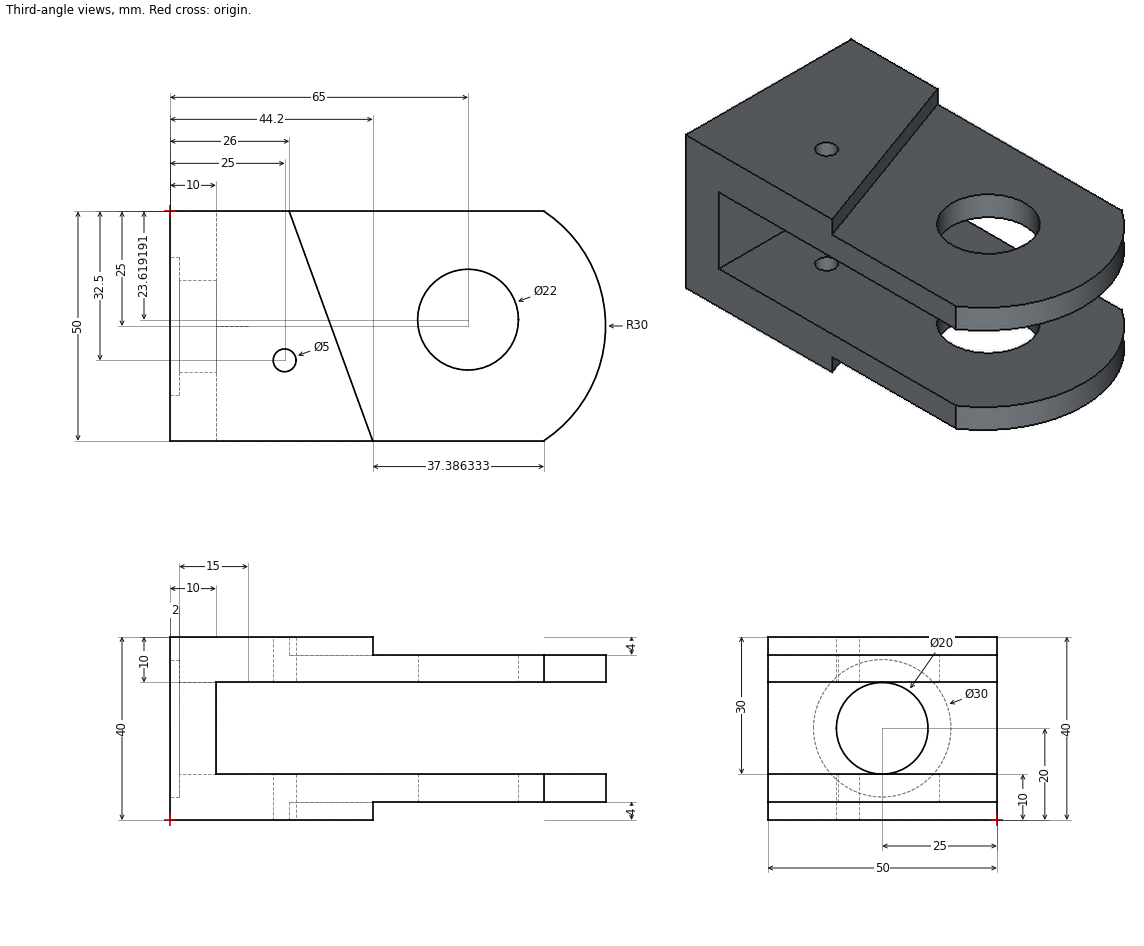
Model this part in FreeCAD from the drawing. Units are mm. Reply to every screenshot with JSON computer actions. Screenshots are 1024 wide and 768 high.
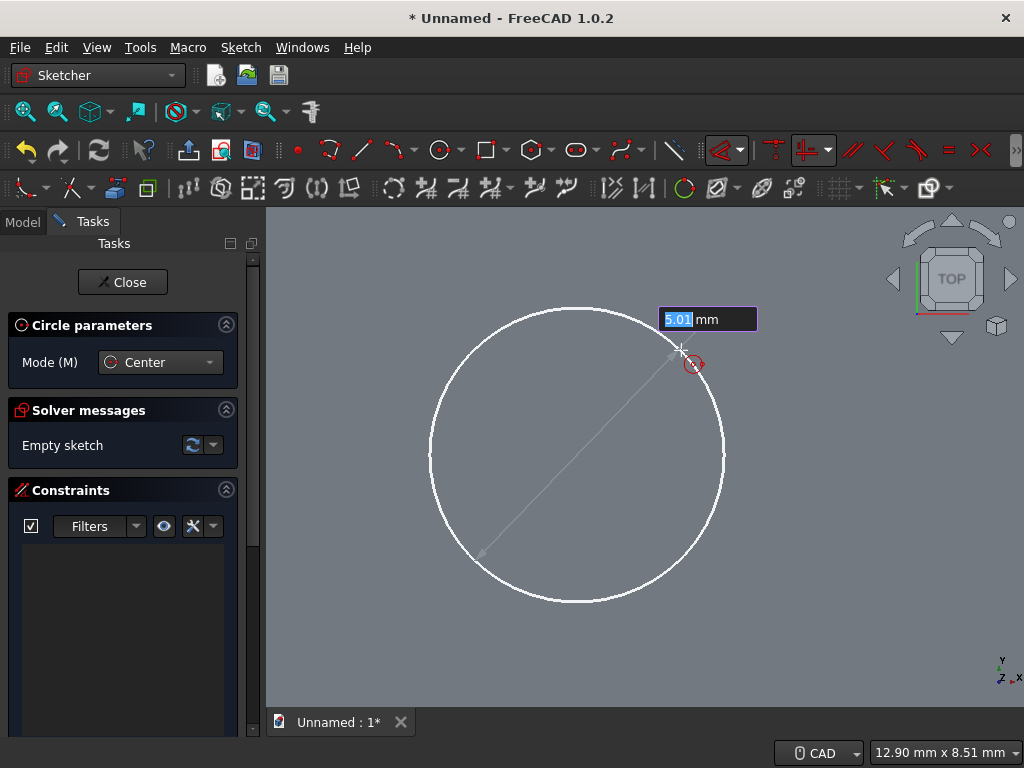
{"action": "type", "text": "5"}
{"action": "key", "text": "Return"}
{"action": "key", "text": "Escape"}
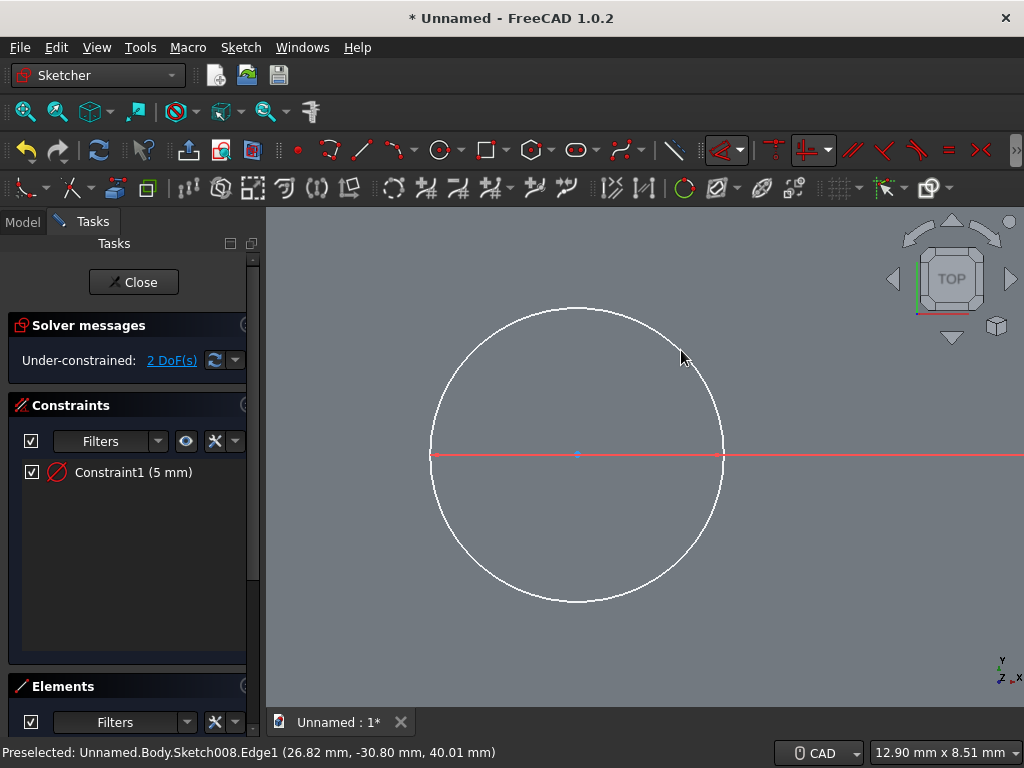
{"action": "left_click", "coordinate": [577, 455]}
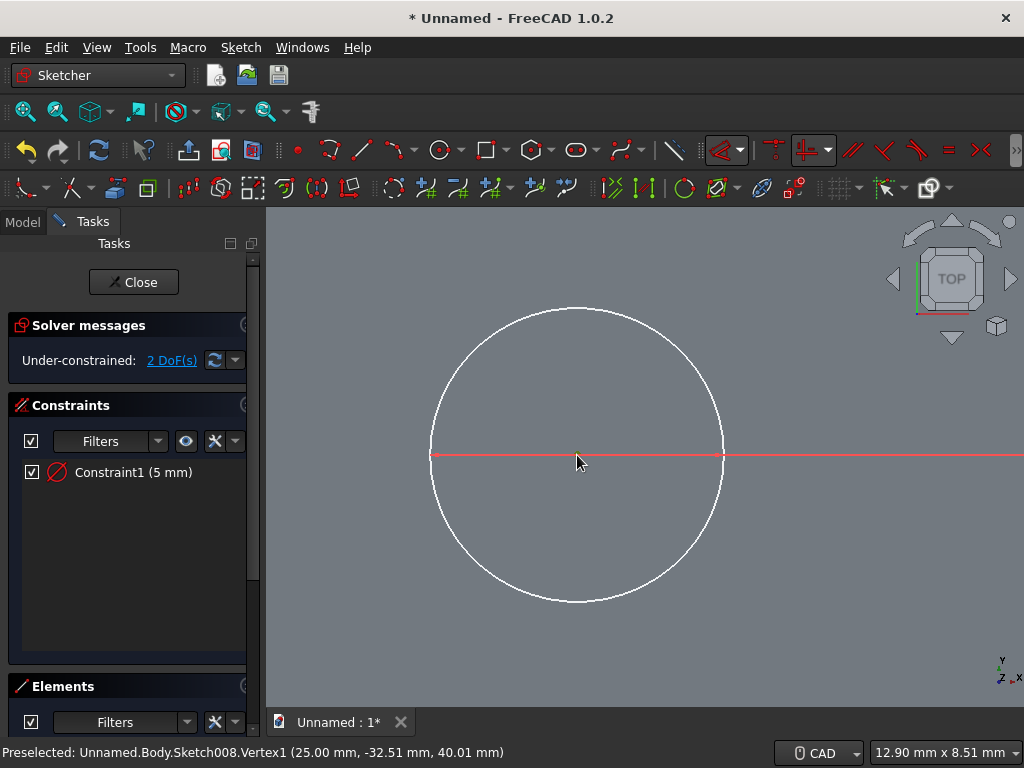
{"action": "key", "text": "l"}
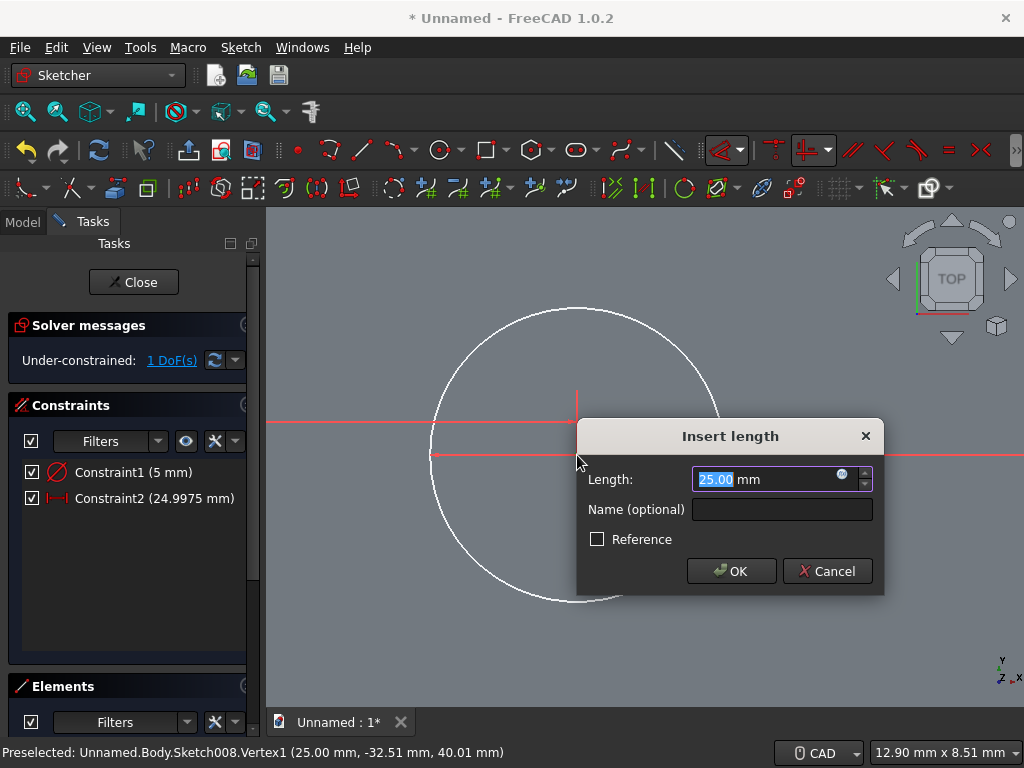
{"action": "type", "text": "25"}
{"action": "key", "text": "Return"}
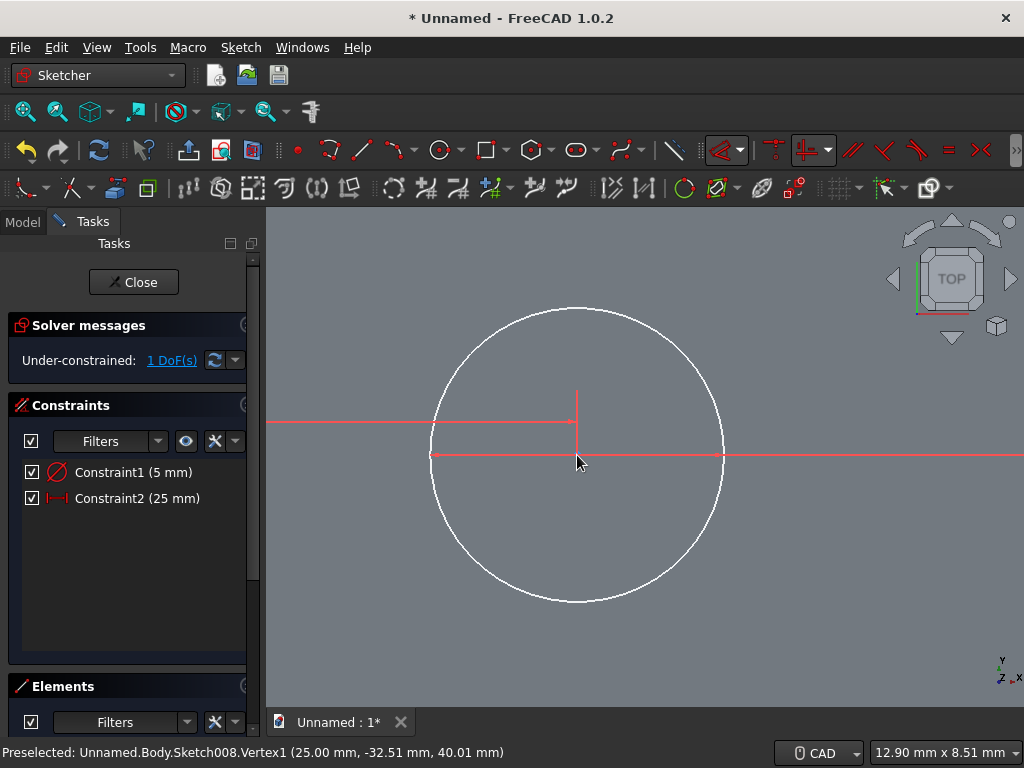
{"action": "left_click", "coordinate": [577, 455]}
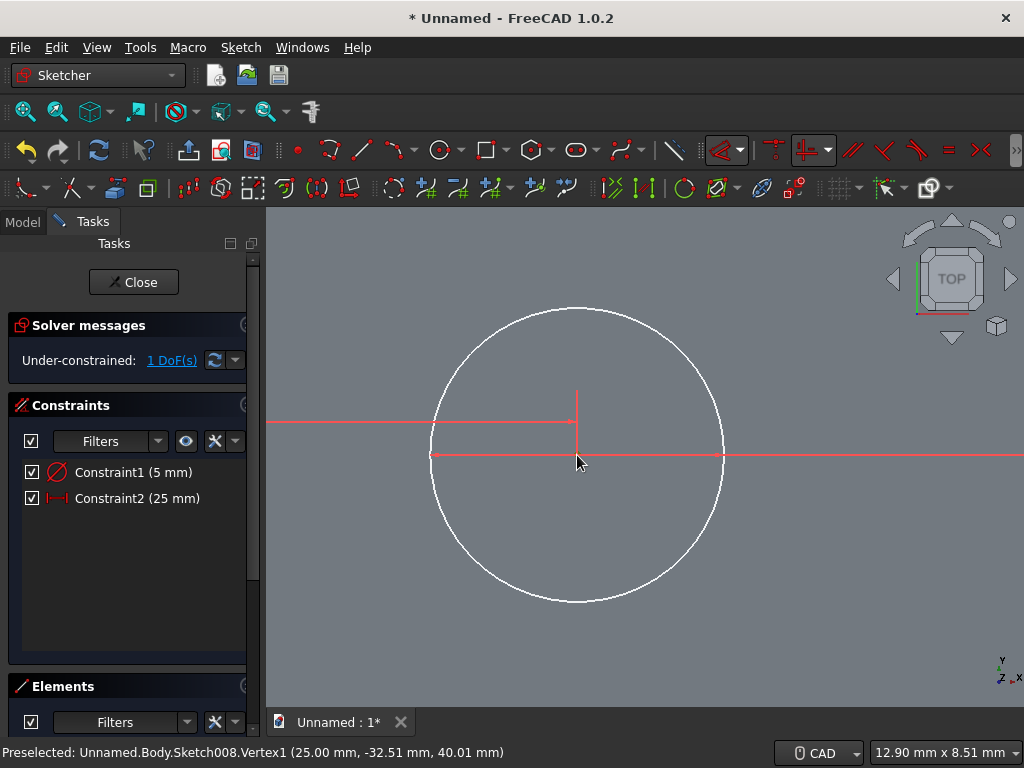
{"action": "key", "text": "i"}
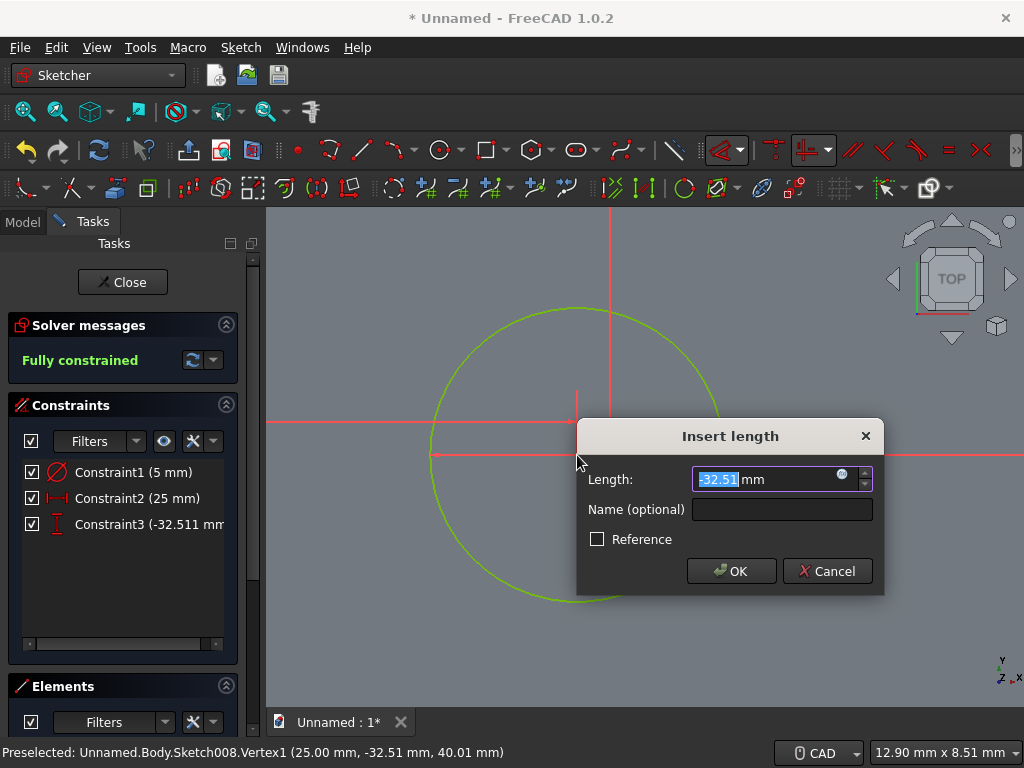
{"action": "type", "text": "-32.5"}
{"action": "key", "text": "Return"}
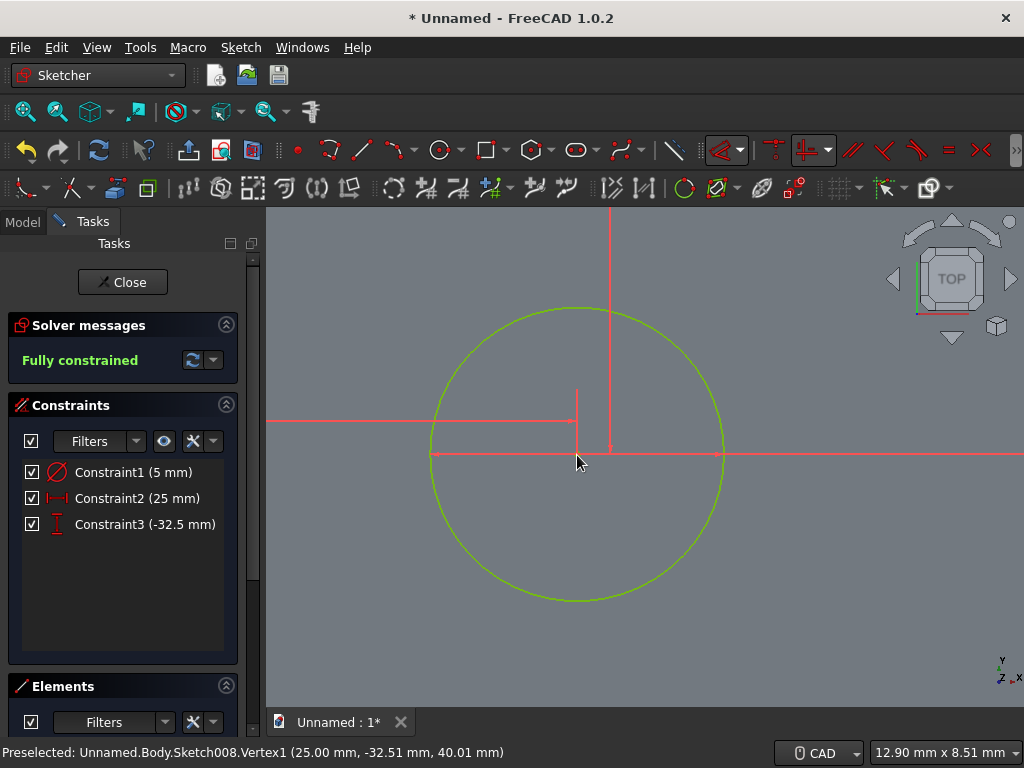
{"action": "left_click", "coordinate": [123, 282]}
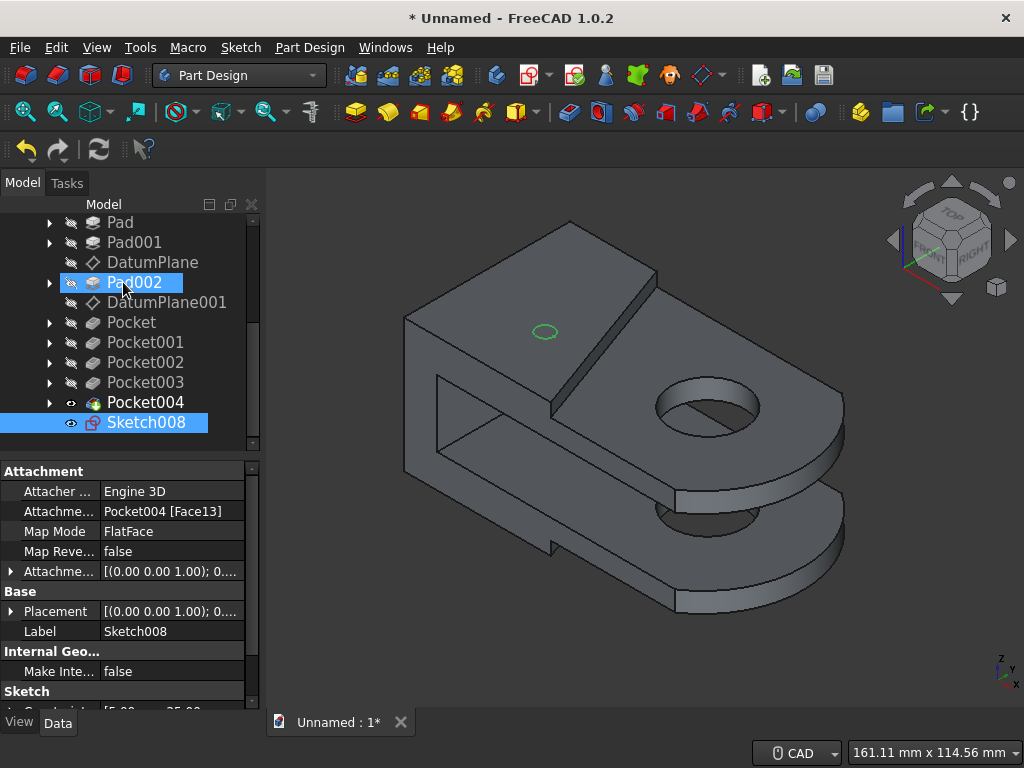
{"action": "left_click", "coordinate": [570, 112]}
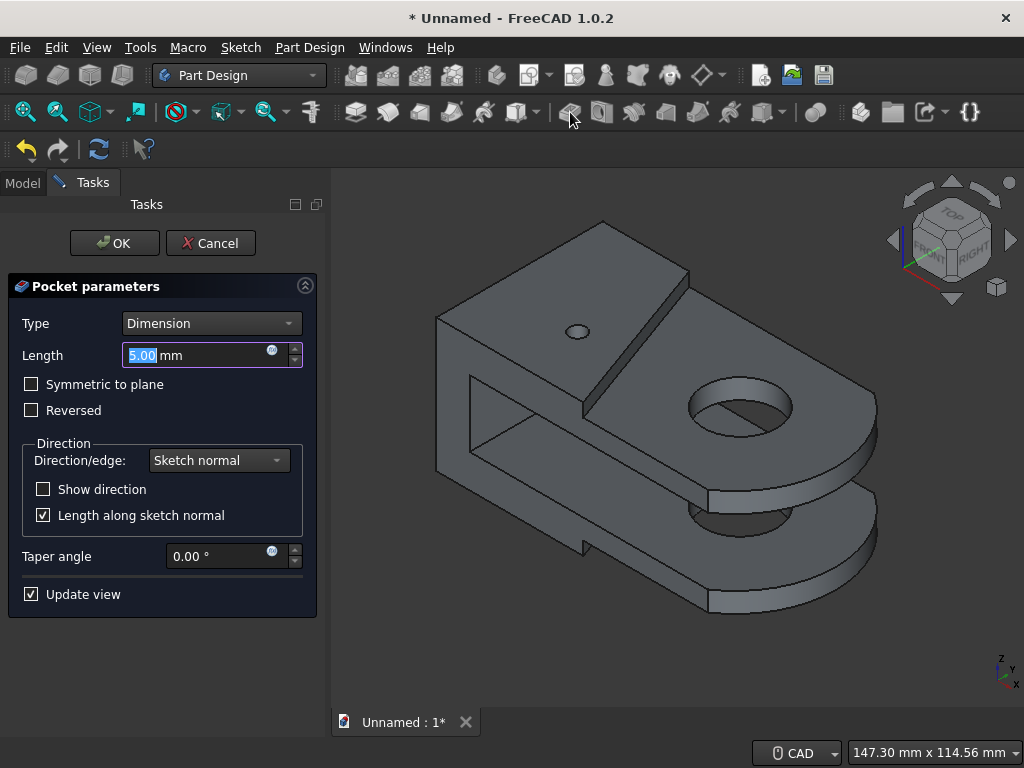
{"action": "type", "text": "40"}
{"action": "key", "text": "Tab"}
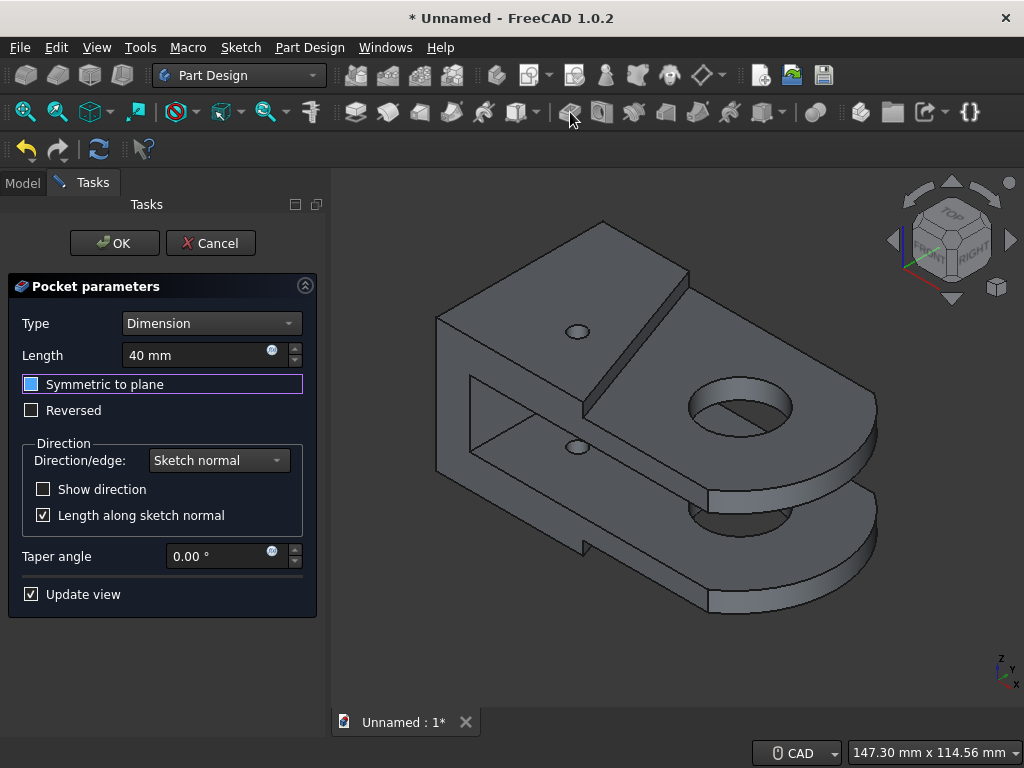
{"action": "left_click", "coordinate": [115, 243]}